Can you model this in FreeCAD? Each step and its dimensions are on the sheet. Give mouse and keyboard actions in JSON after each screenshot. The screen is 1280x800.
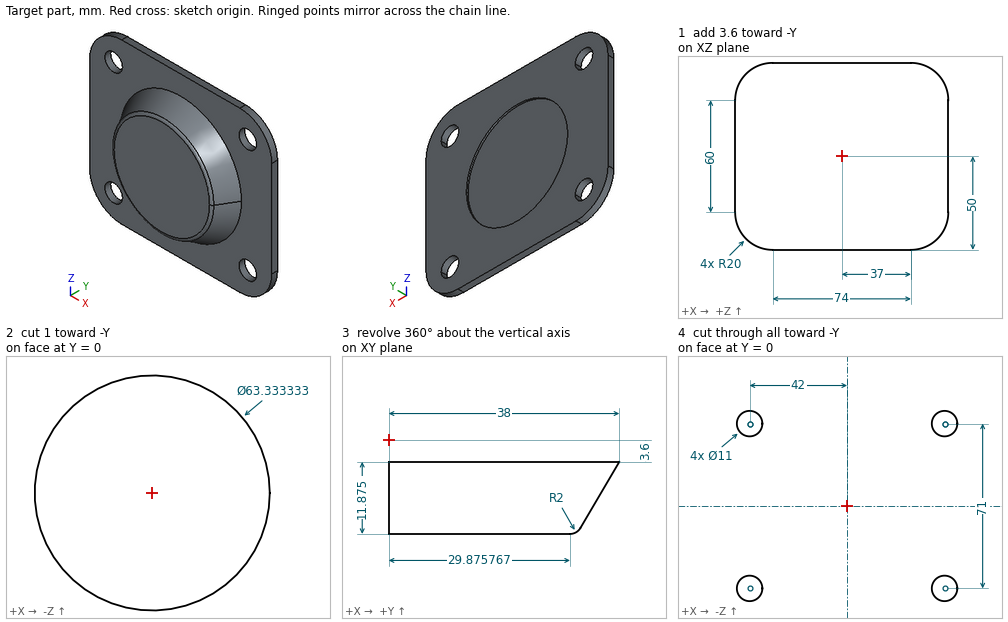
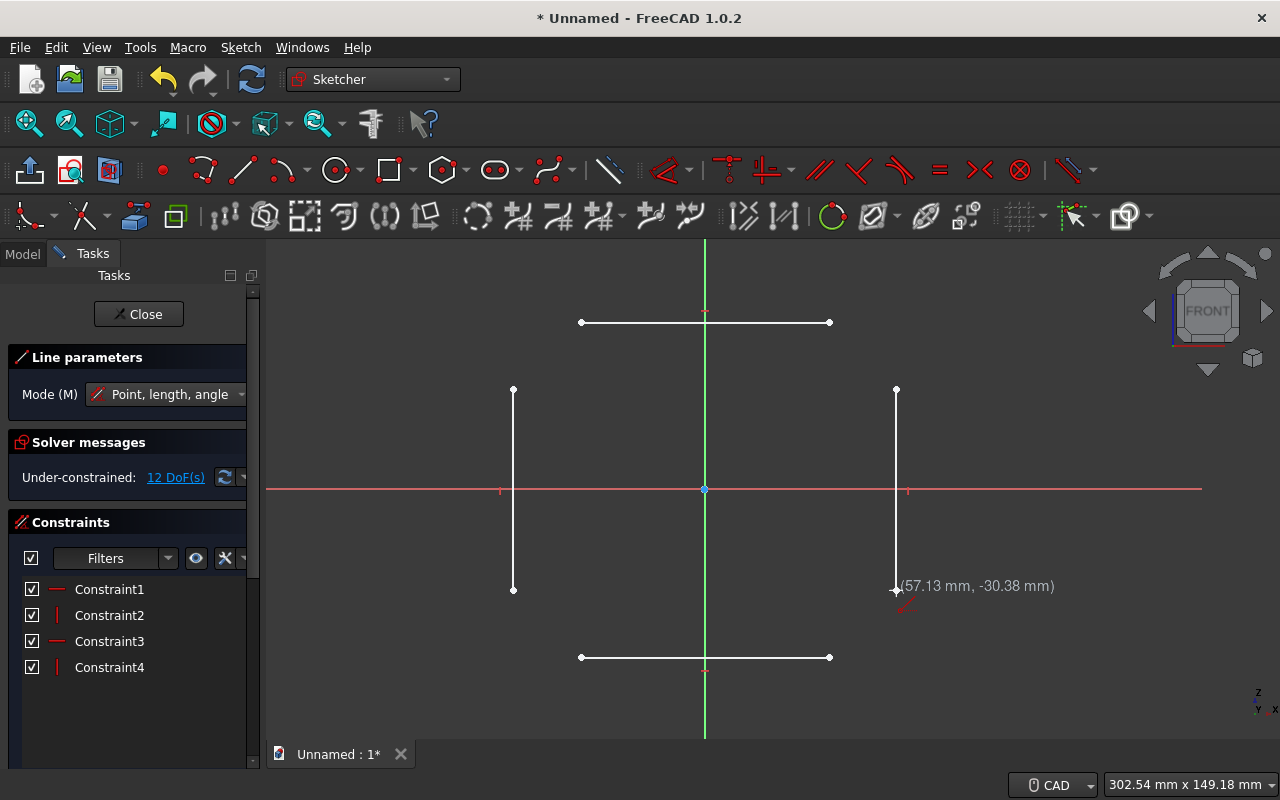
{"action": "key", "text": "g 3 a"}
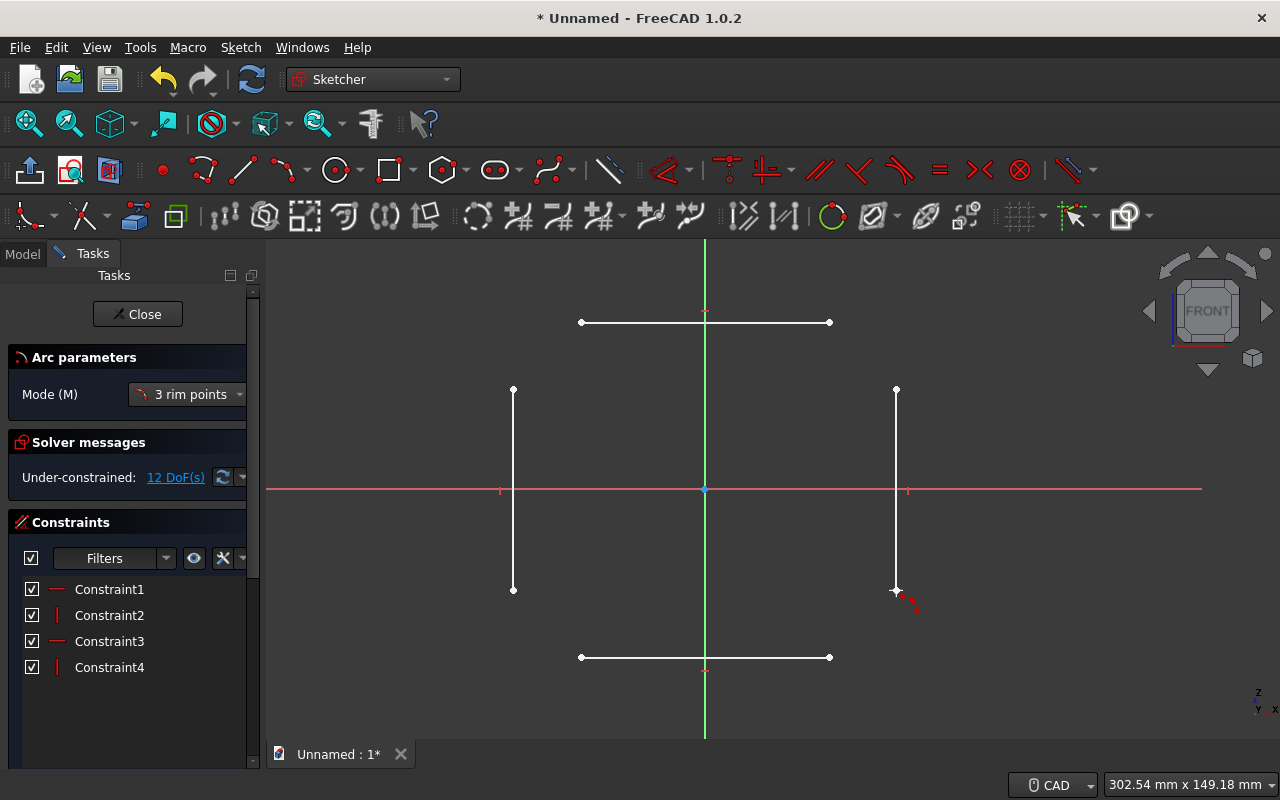
{"action": "left_click", "coordinate": [581, 658]}
{"action": "left_click", "coordinate": [513, 591]}
{"action": "left_click", "coordinate": [533, 637]}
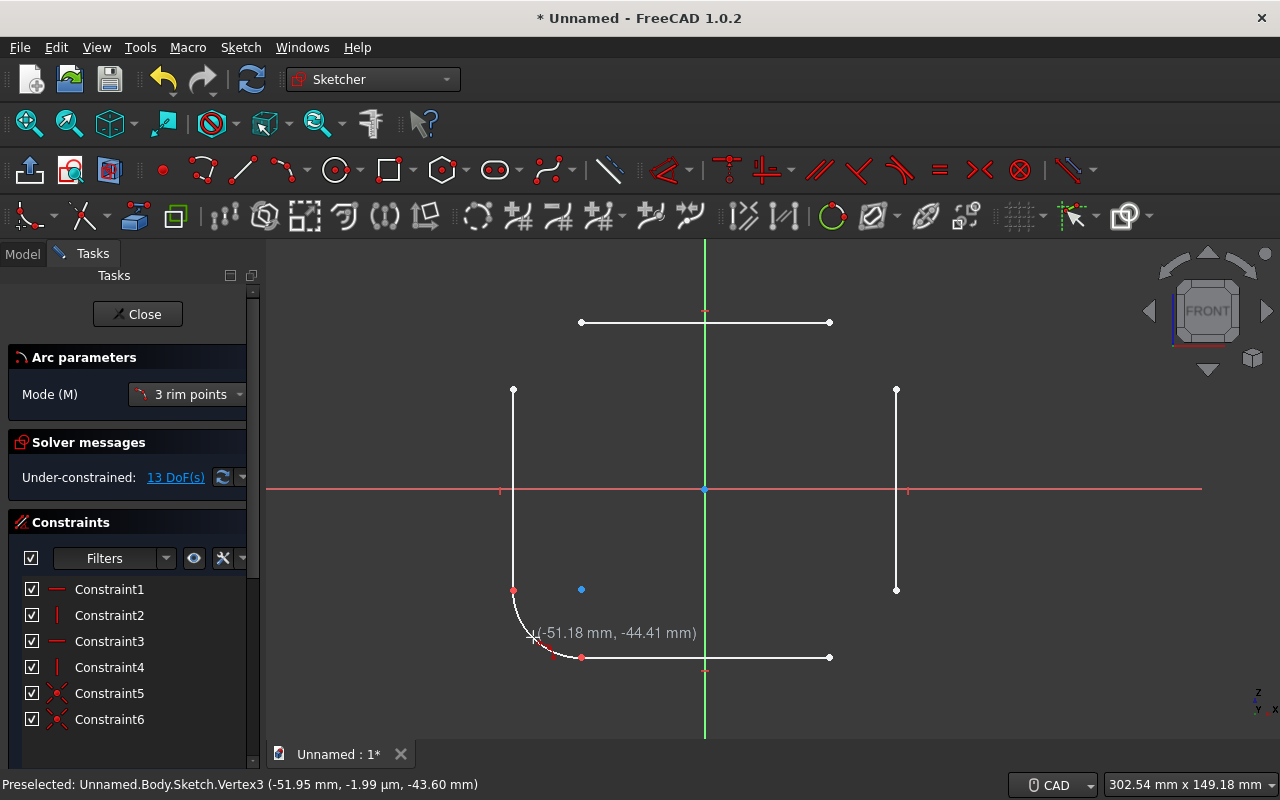
{"action": "left_click", "coordinate": [513, 390]}
{"action": "left_click", "coordinate": [581, 323]}
{"action": "left_click", "coordinate": [533, 341]}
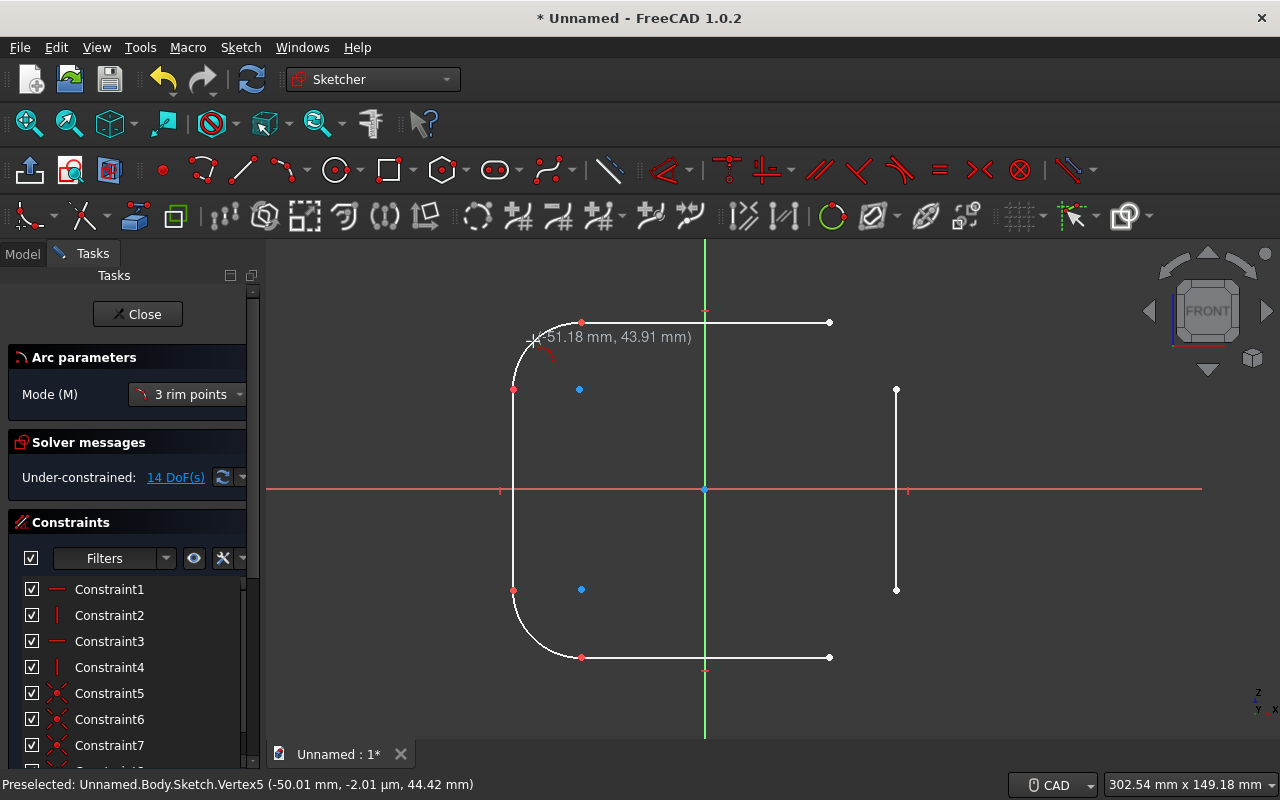
{"action": "left_click", "coordinate": [829, 323]}
{"action": "left_click", "coordinate": [896, 390]}
{"action": "left_click", "coordinate": [876, 341]}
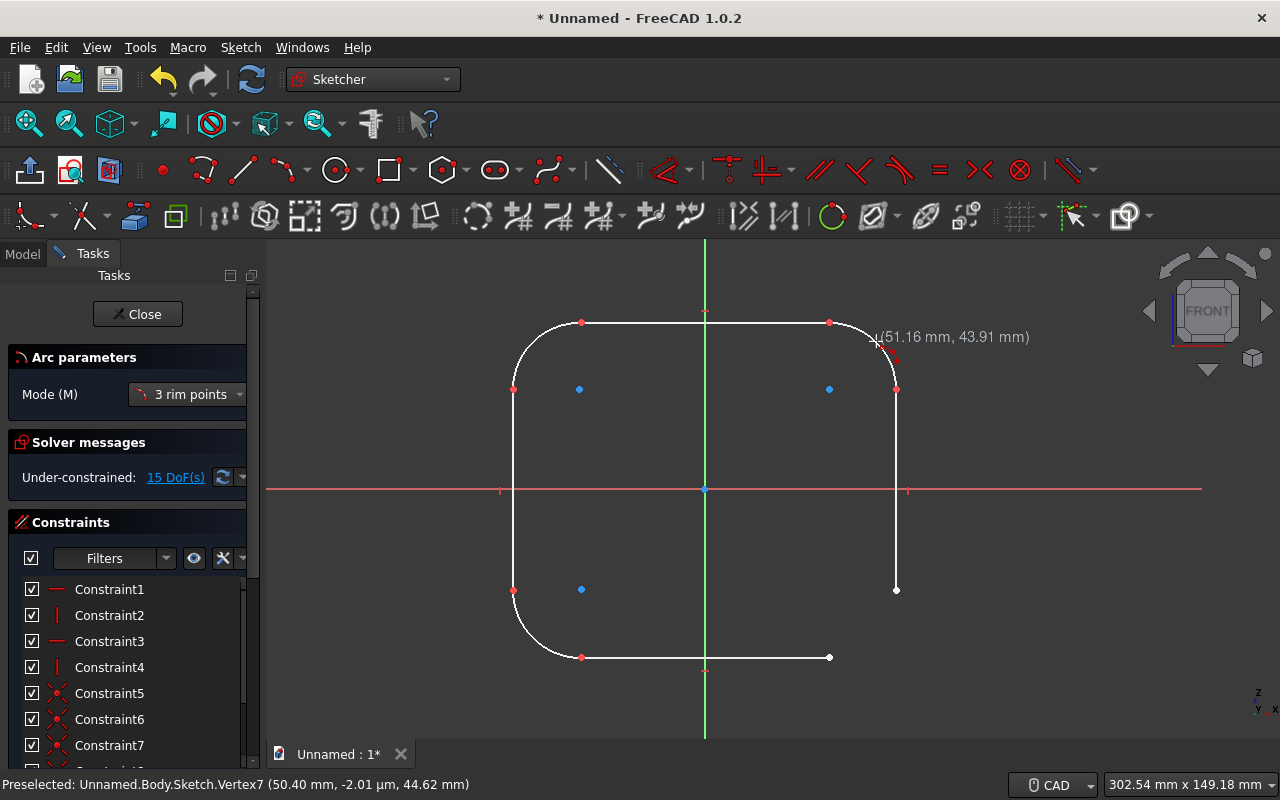
{"action": "left_click", "coordinate": [896, 591]}
{"action": "left_click", "coordinate": [829, 658]}
{"action": "left_click", "coordinate": [876, 637]}
{"action": "key", "text": "Escape"}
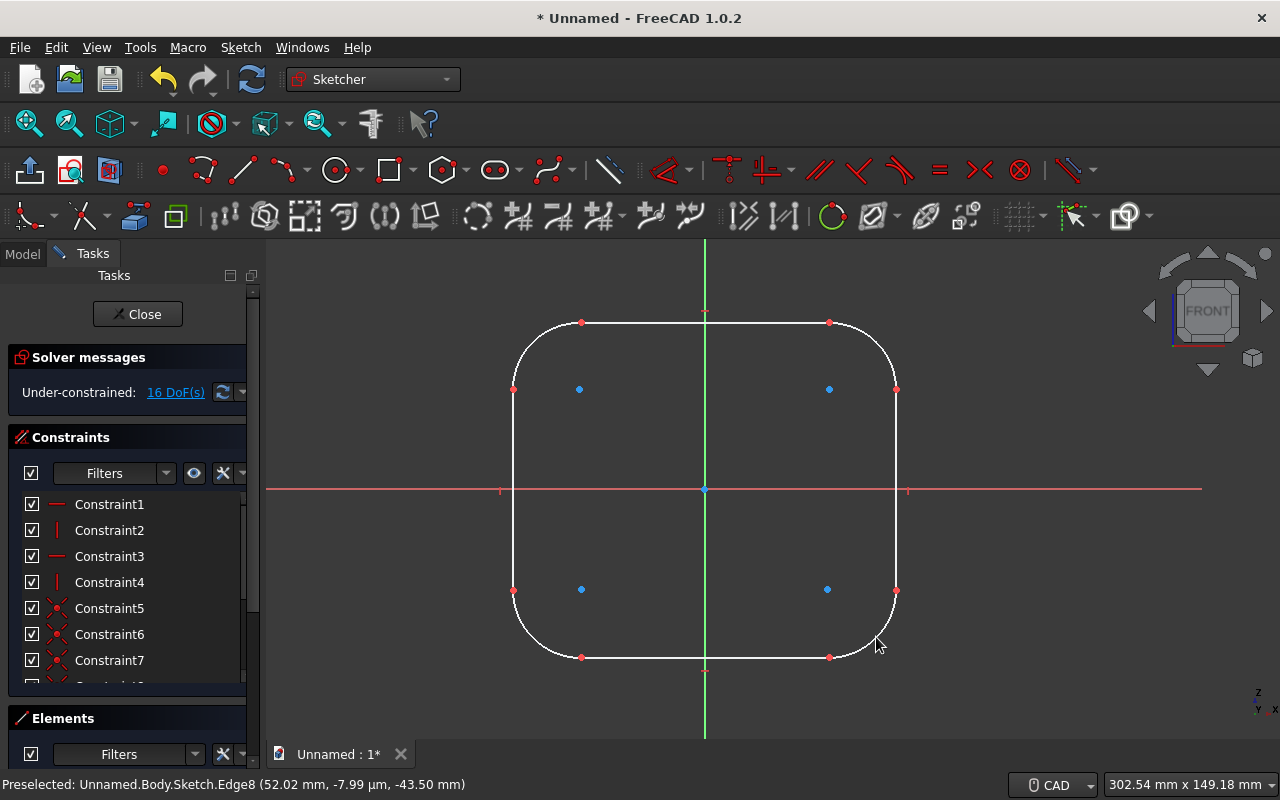
{"action": "left_click", "coordinate": [755, 658]}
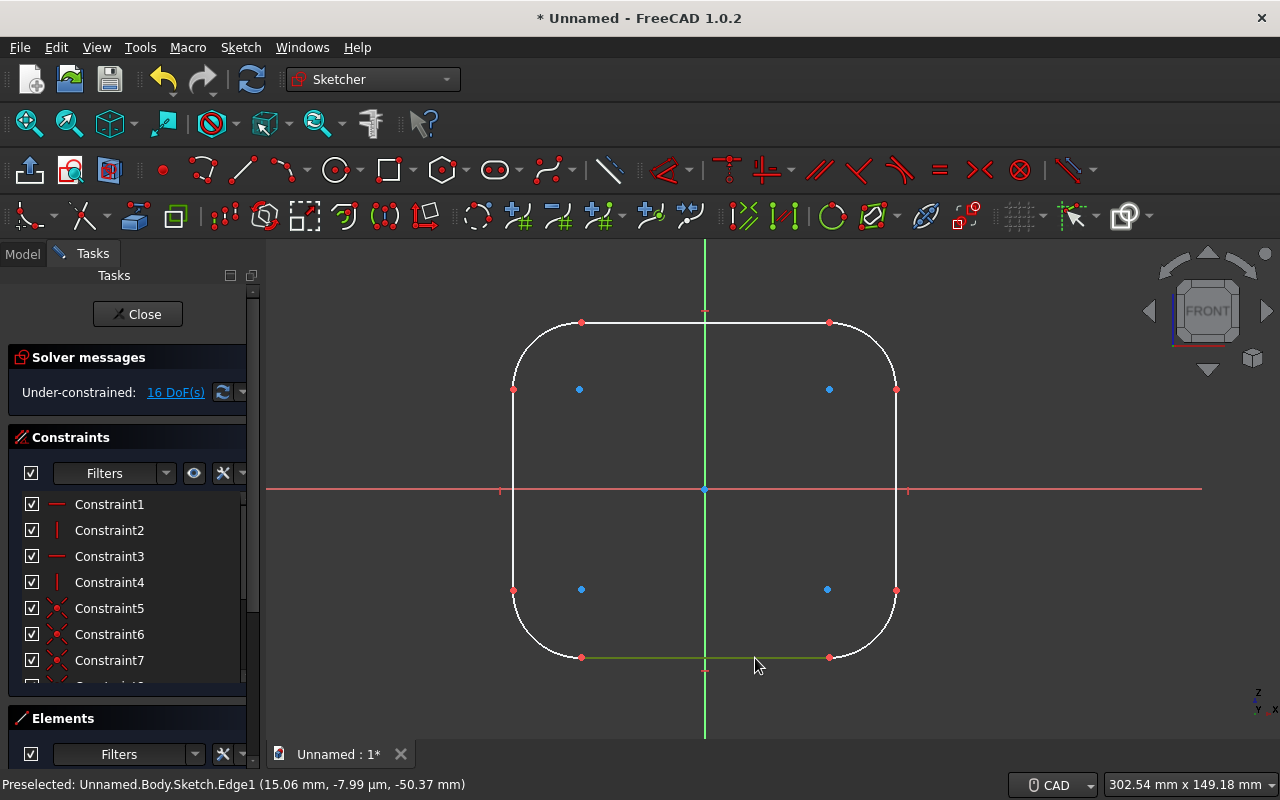
{"action": "left_click", "coordinate": [521, 621]}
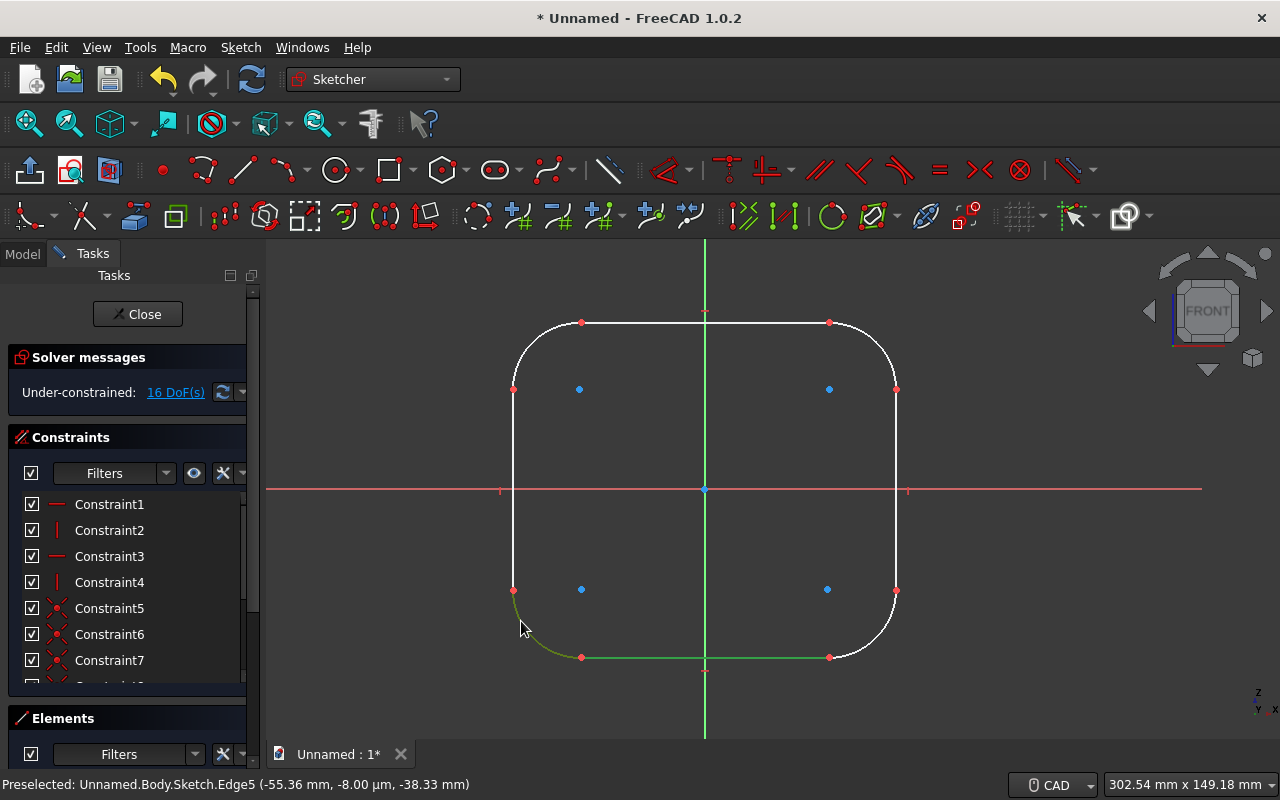
{"action": "left_click", "coordinate": [900, 170]}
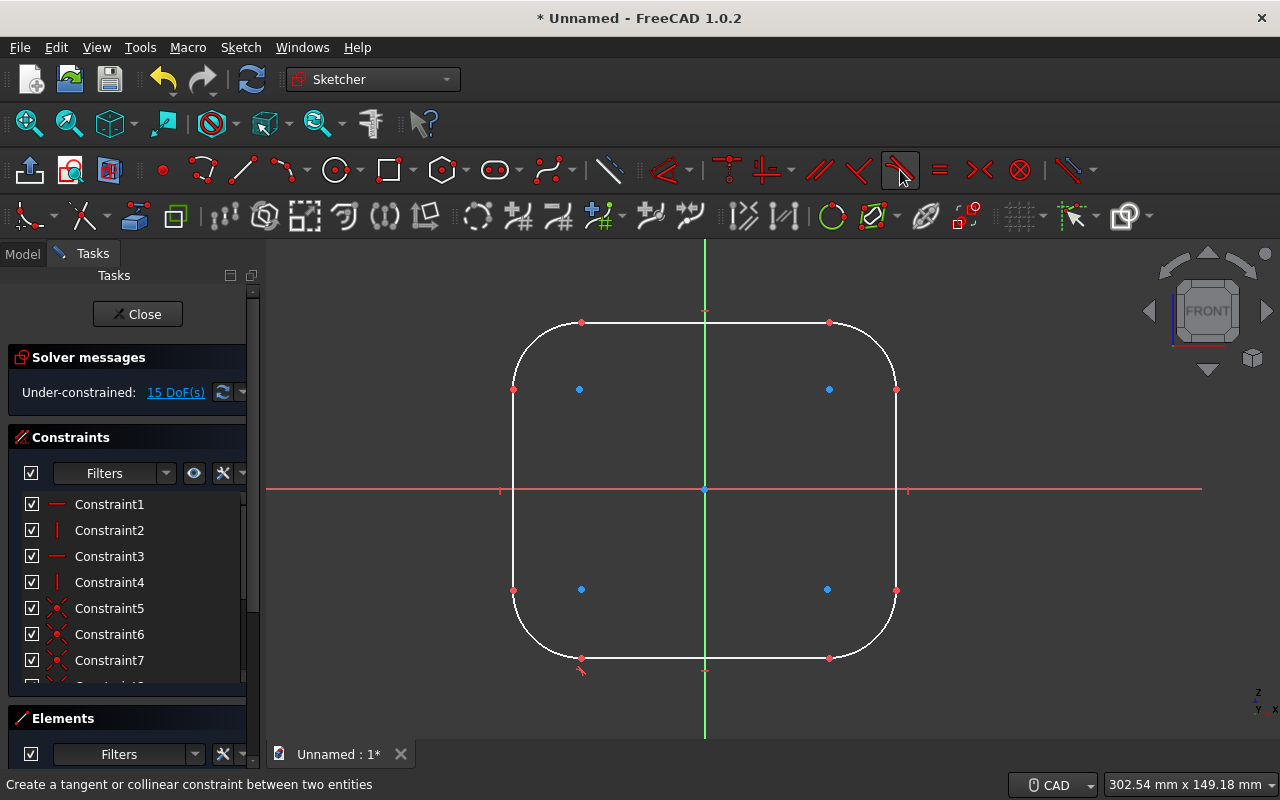
{"action": "left_click", "coordinate": [755, 658]}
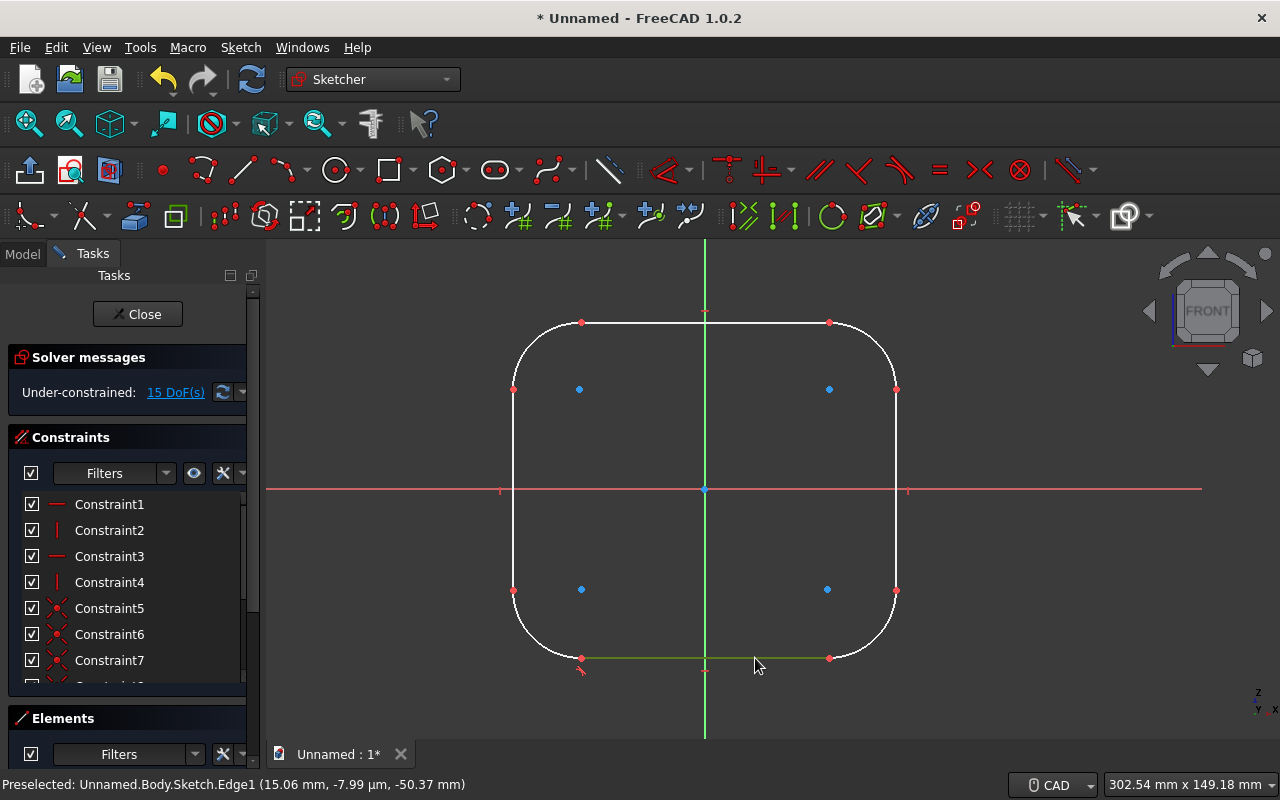
{"action": "left_click", "coordinate": [859, 650]}